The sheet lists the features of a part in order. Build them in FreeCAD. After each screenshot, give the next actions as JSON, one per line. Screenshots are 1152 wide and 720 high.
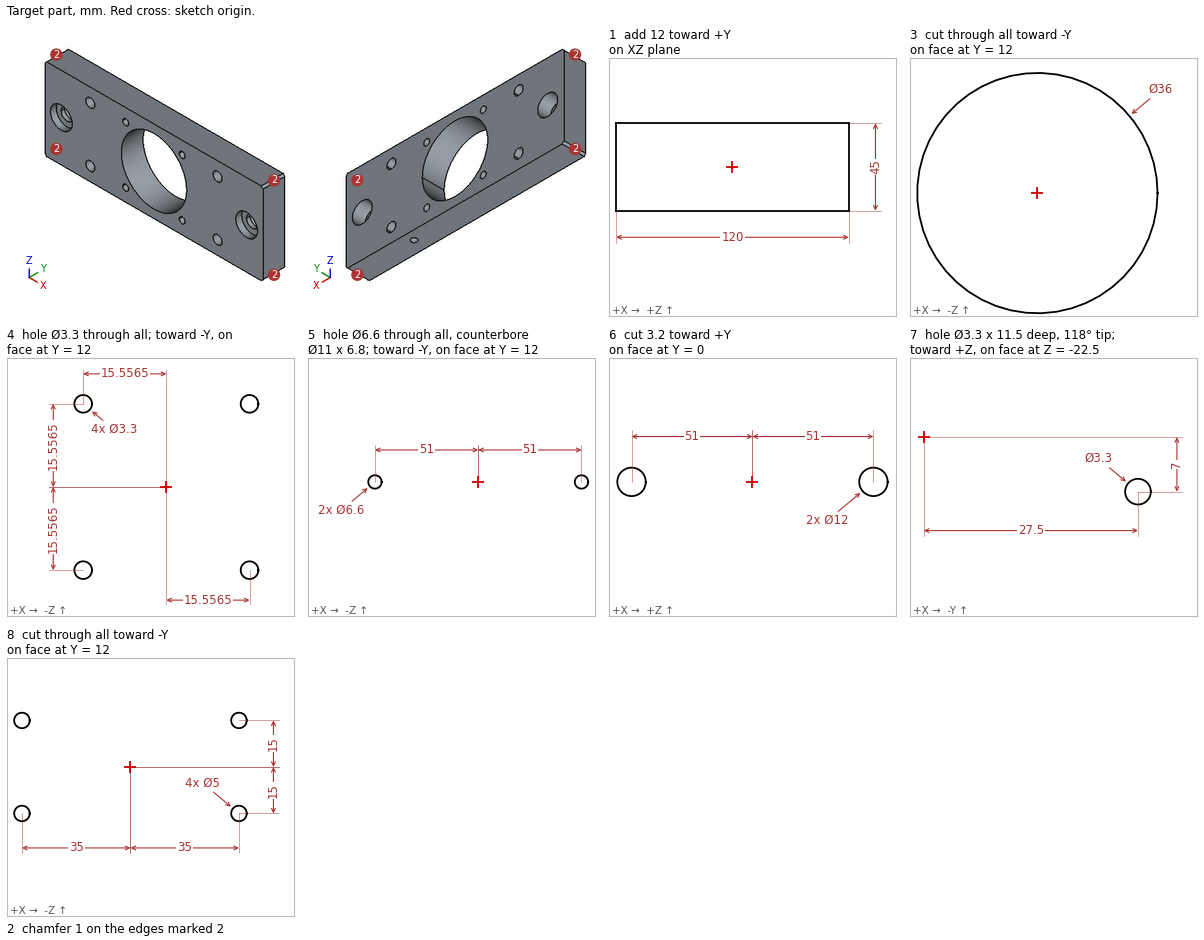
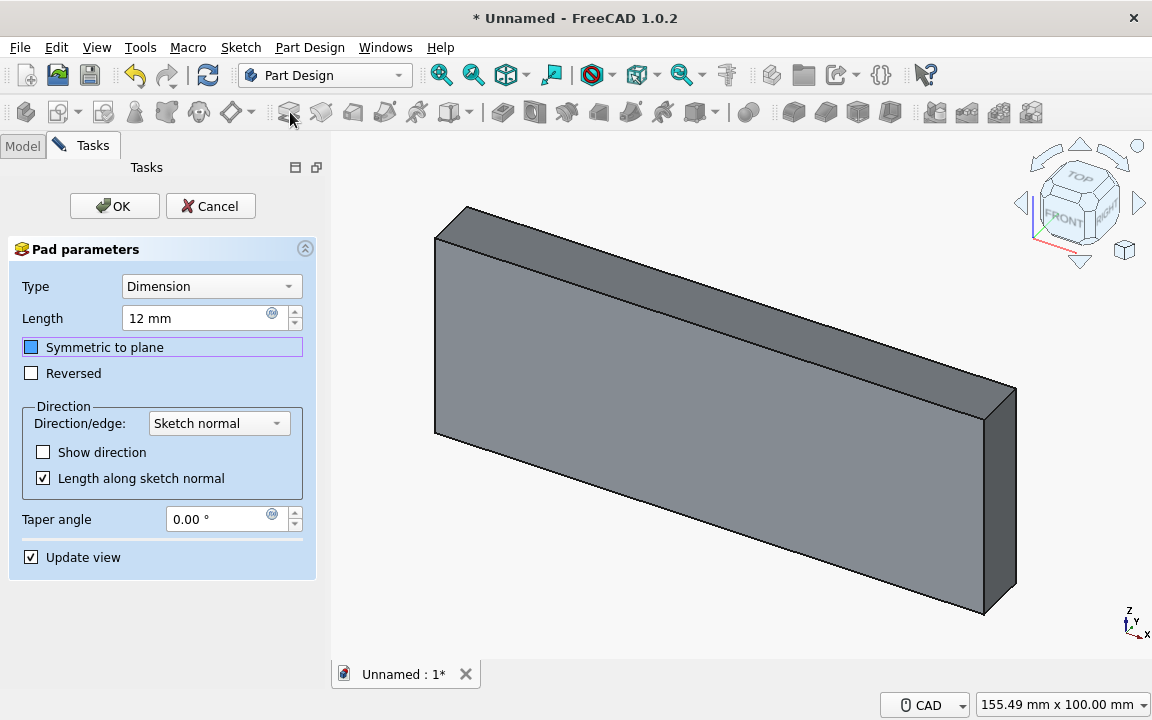
{"action": "left_click", "coordinate": [30, 373]}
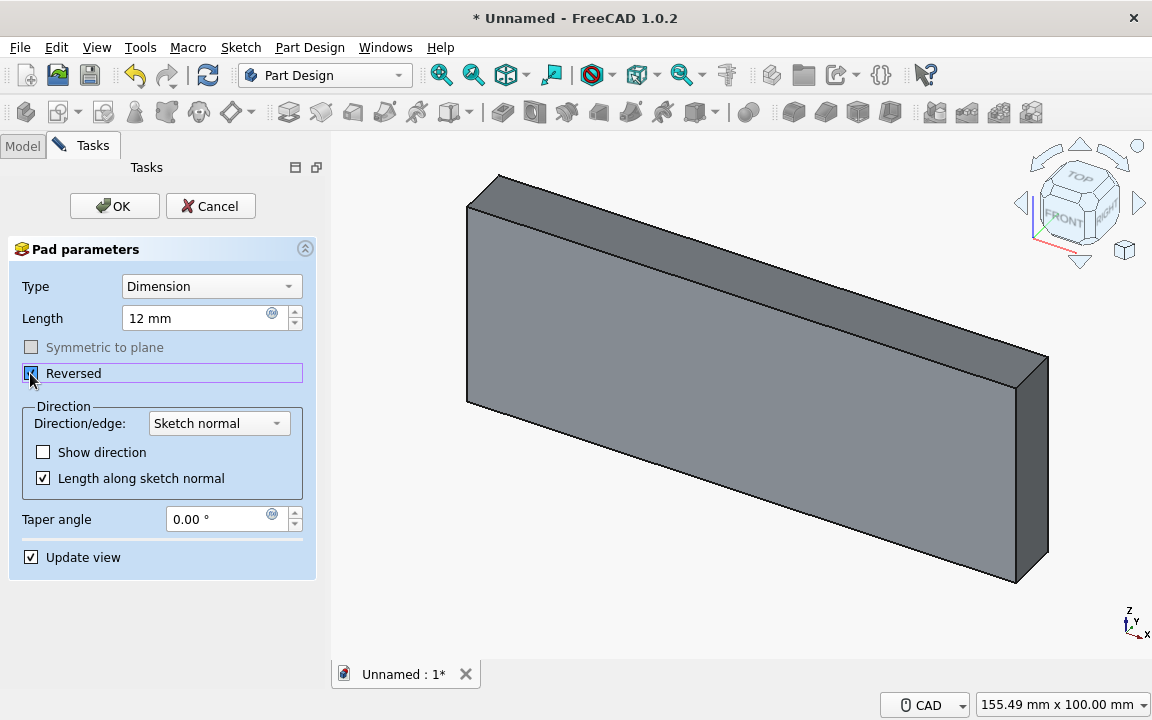
{"action": "left_click", "coordinate": [115, 206]}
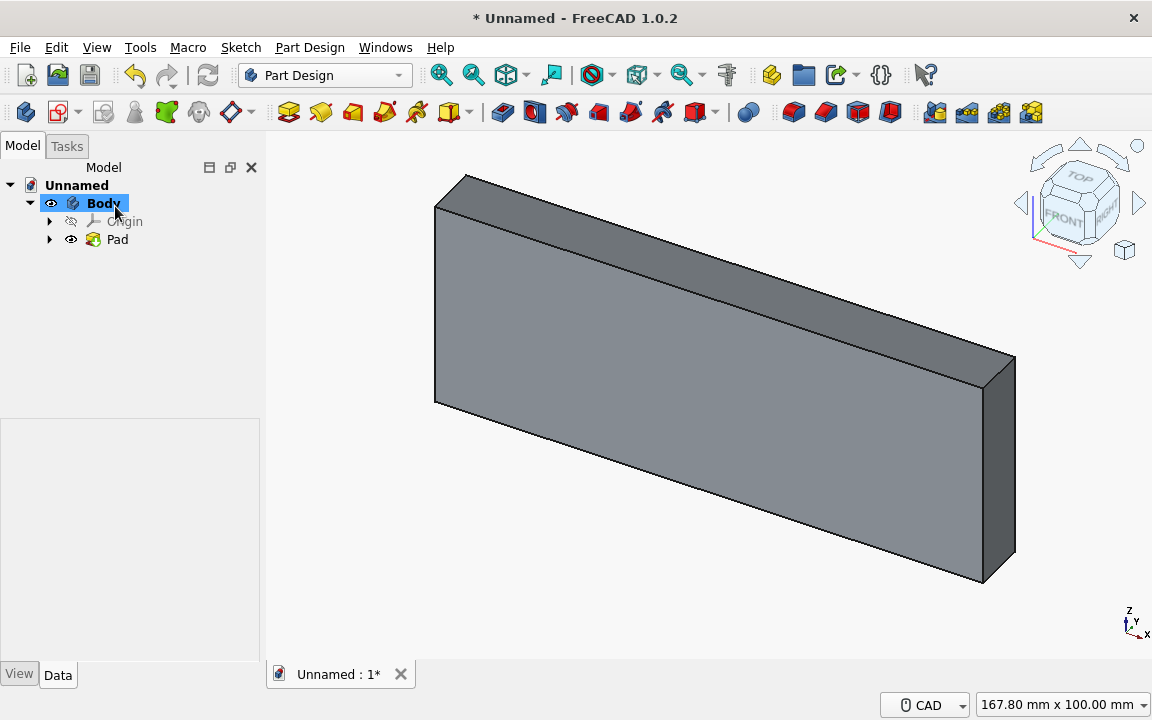
{"action": "left_click", "coordinate": [999, 372]}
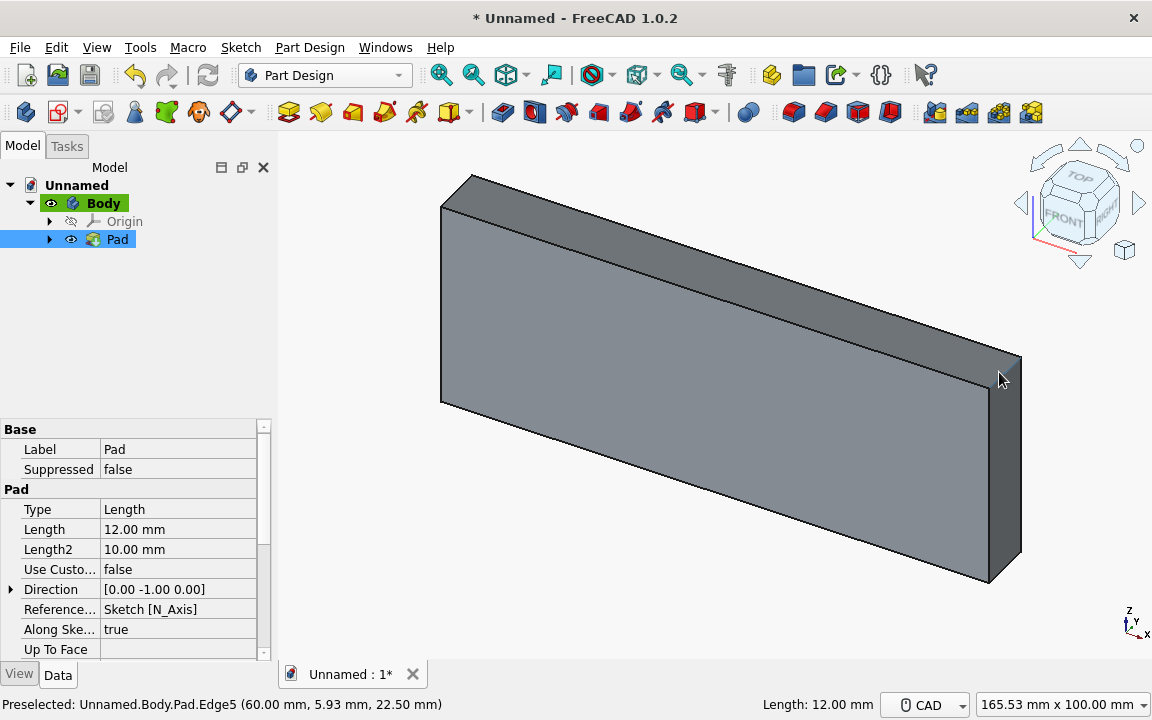
{"action": "key", "text": "0"}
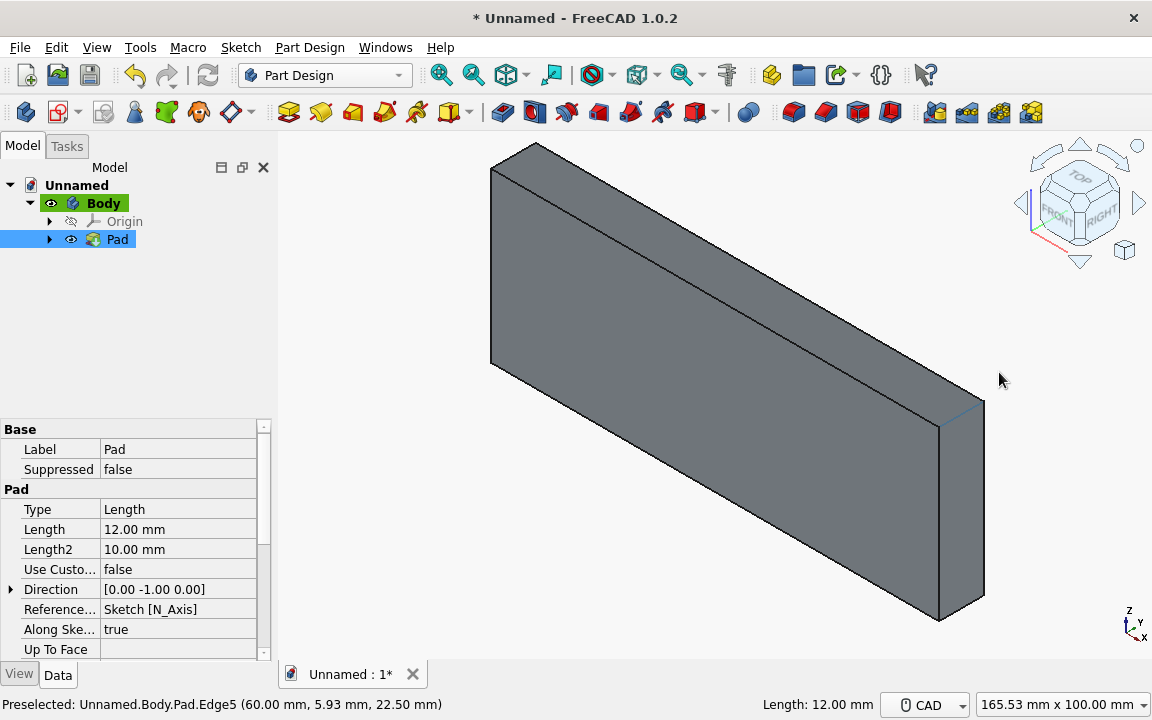
{"action": "key", "text": "2"}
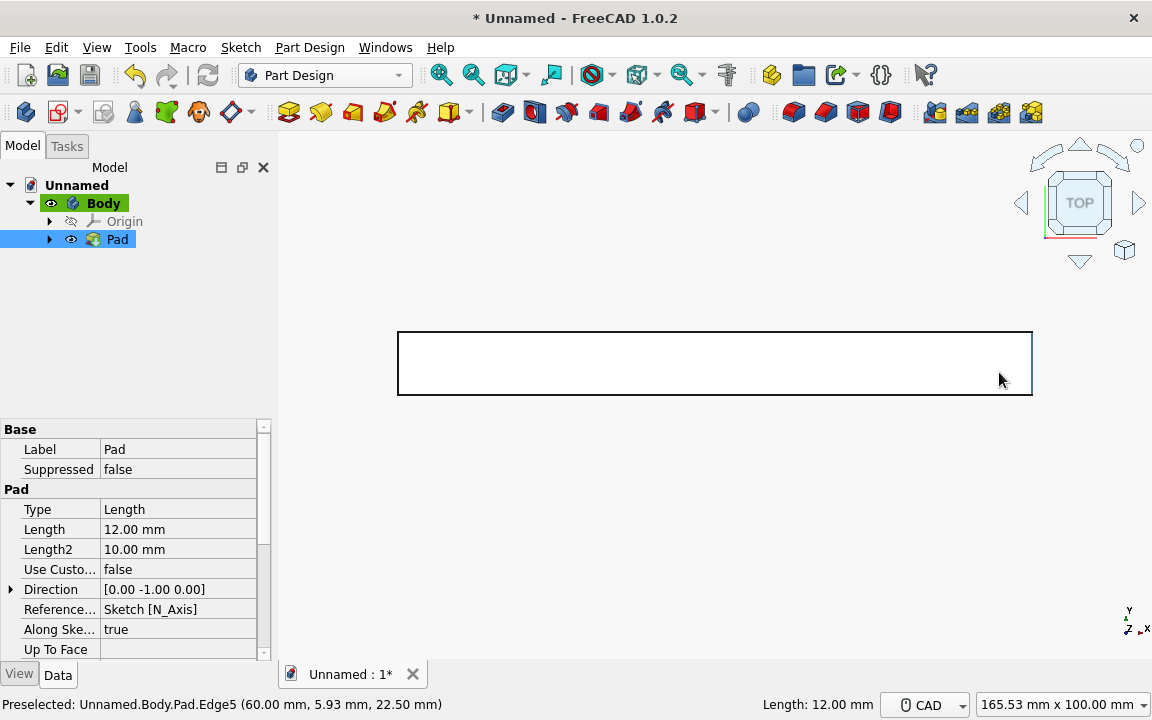
{"action": "left_click", "coordinate": [398, 362], "text": "ctrl"}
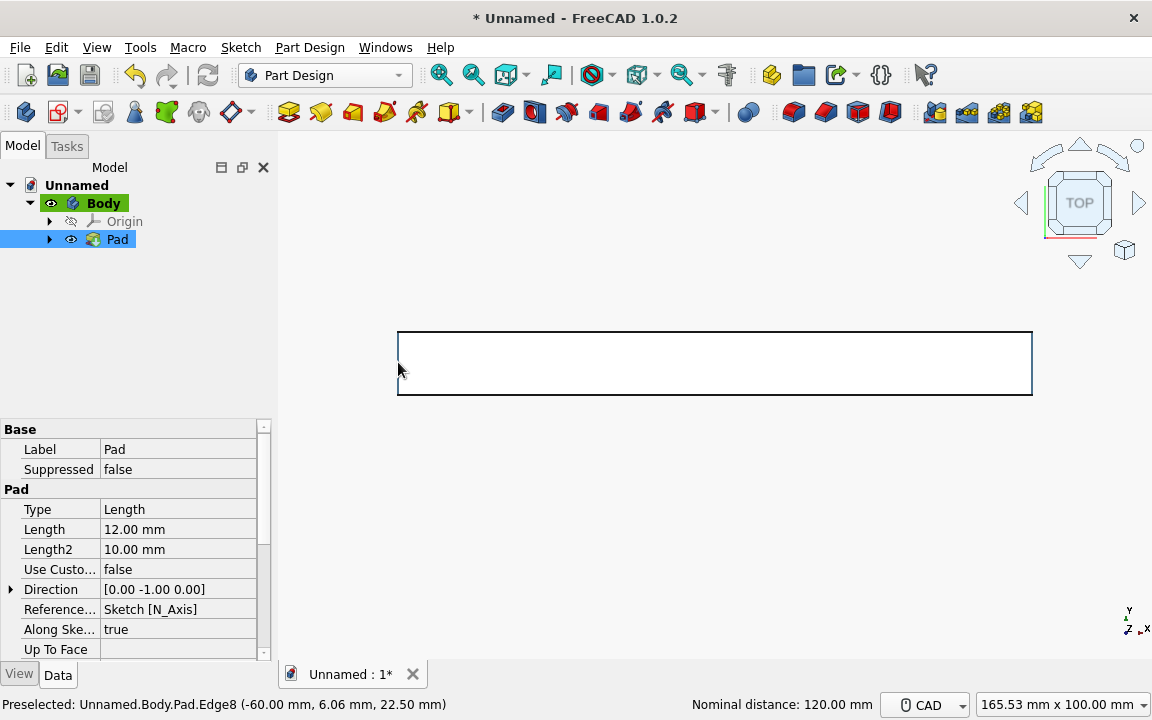
{"action": "key", "text": "1"}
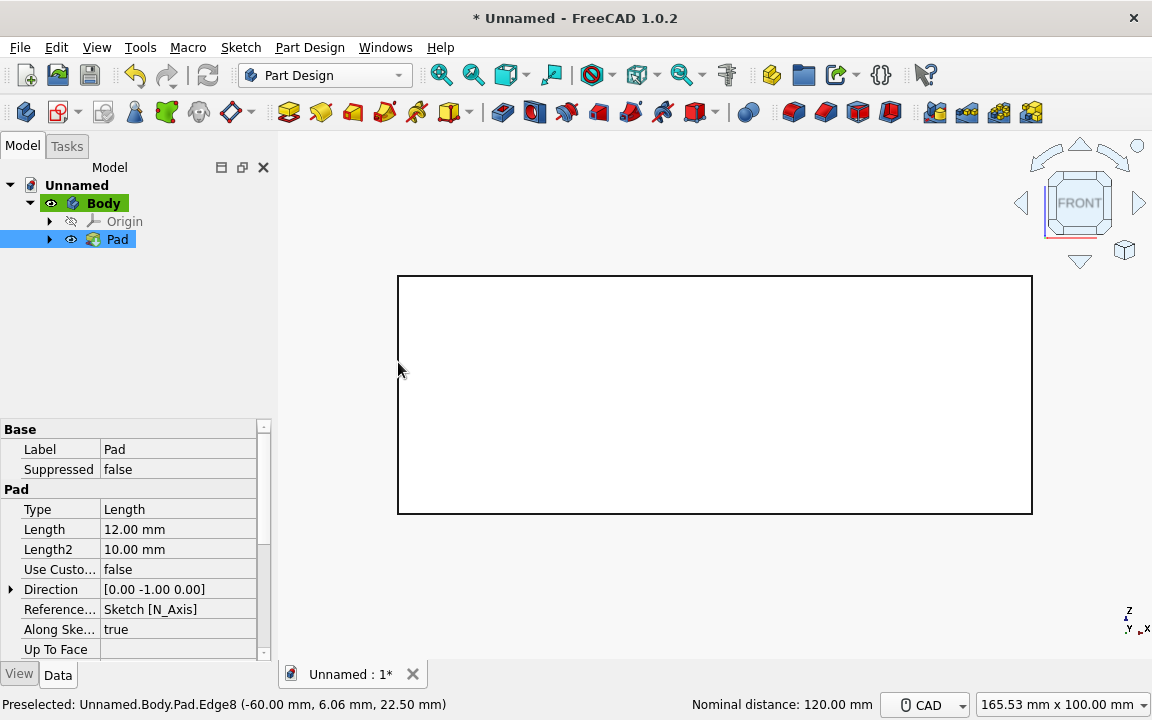
{"action": "key", "text": "3"}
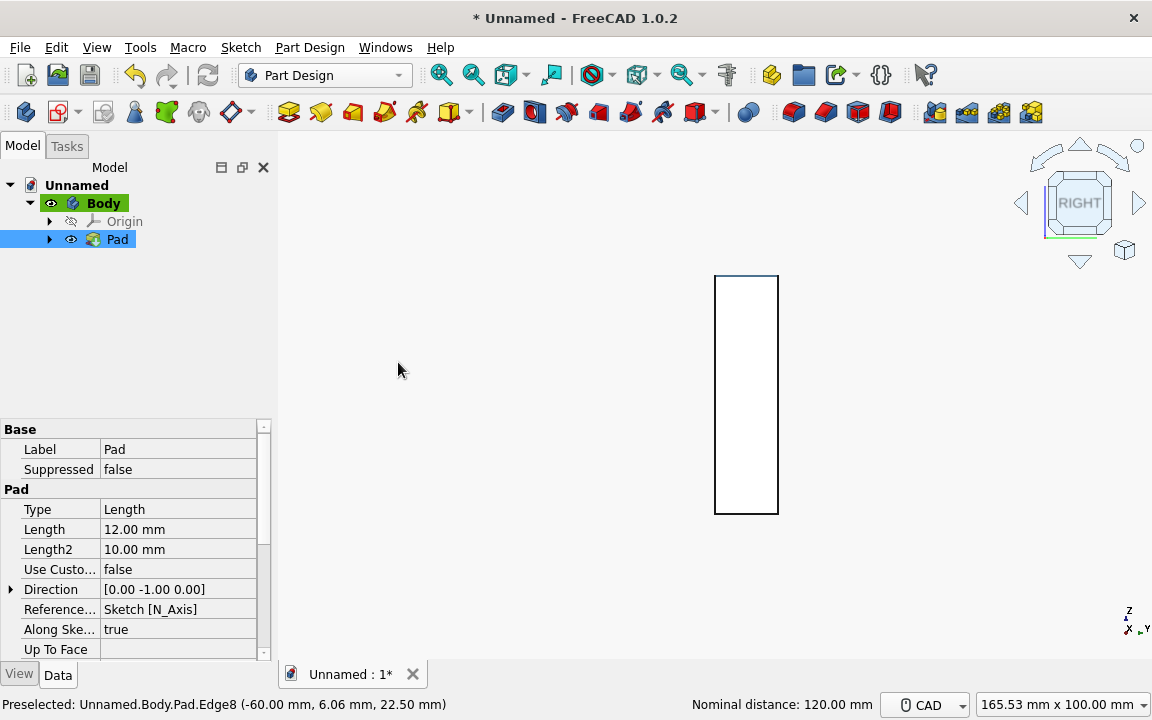
{"action": "left_click", "coordinate": [747, 513], "text": "ctrl"}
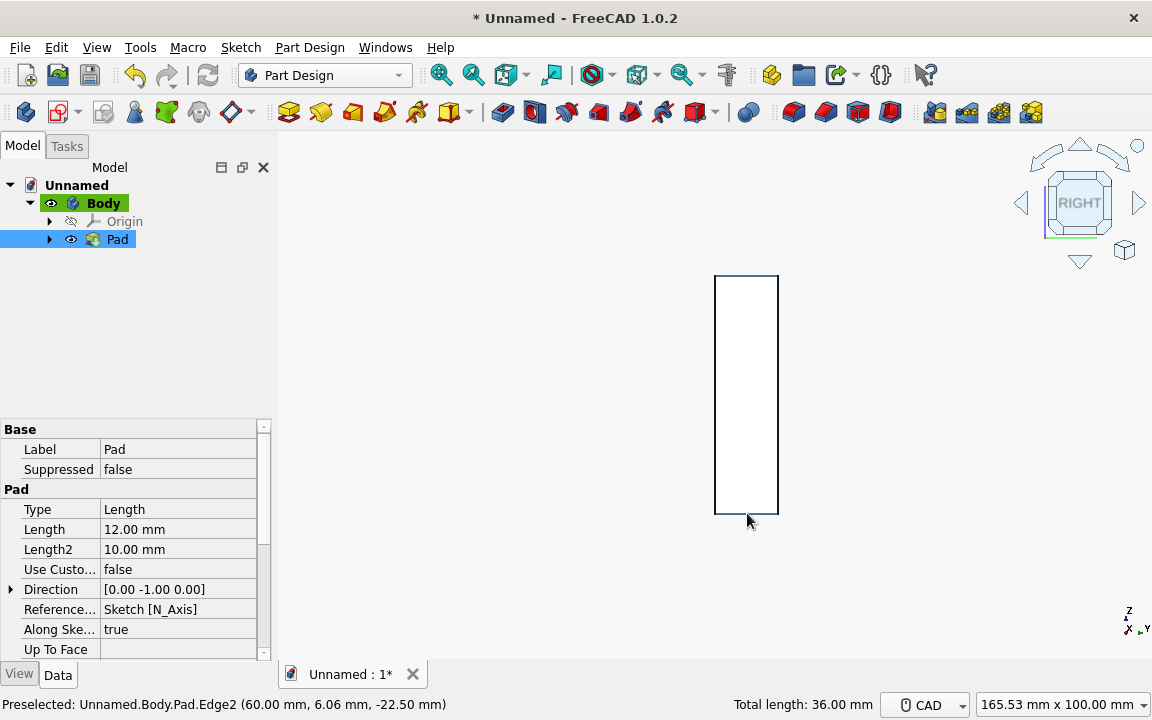
{"action": "key", "text": "5"}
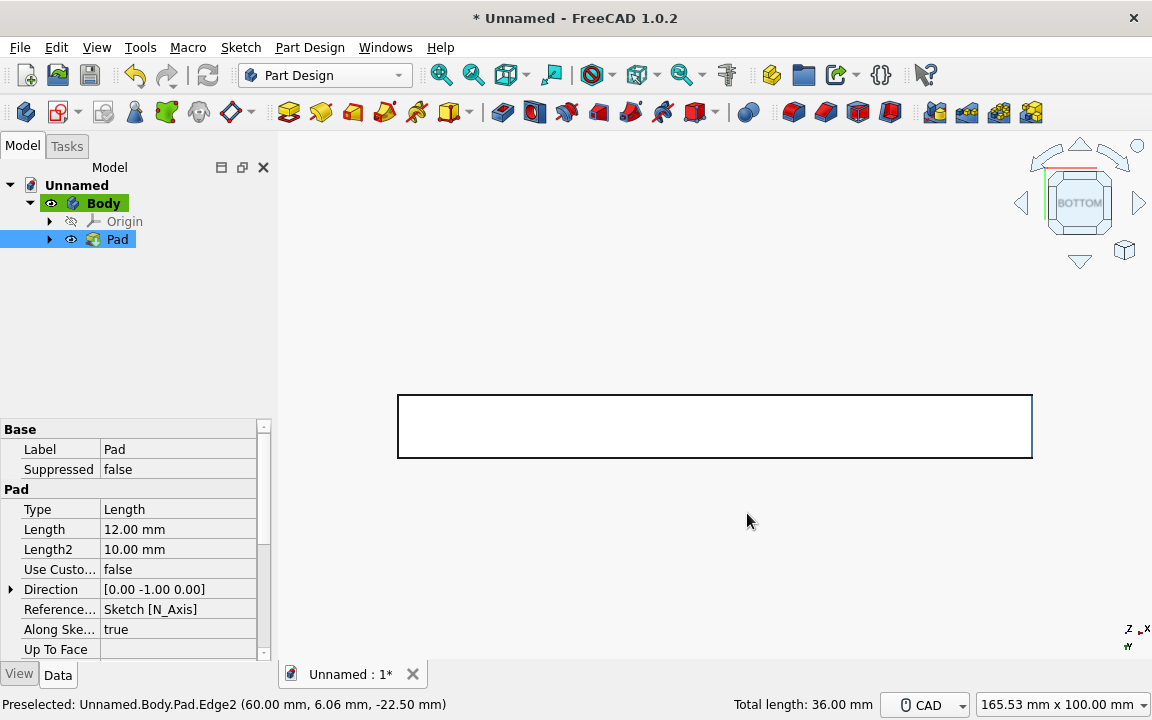
{"action": "left_click", "coordinate": [398, 426], "text": "ctrl"}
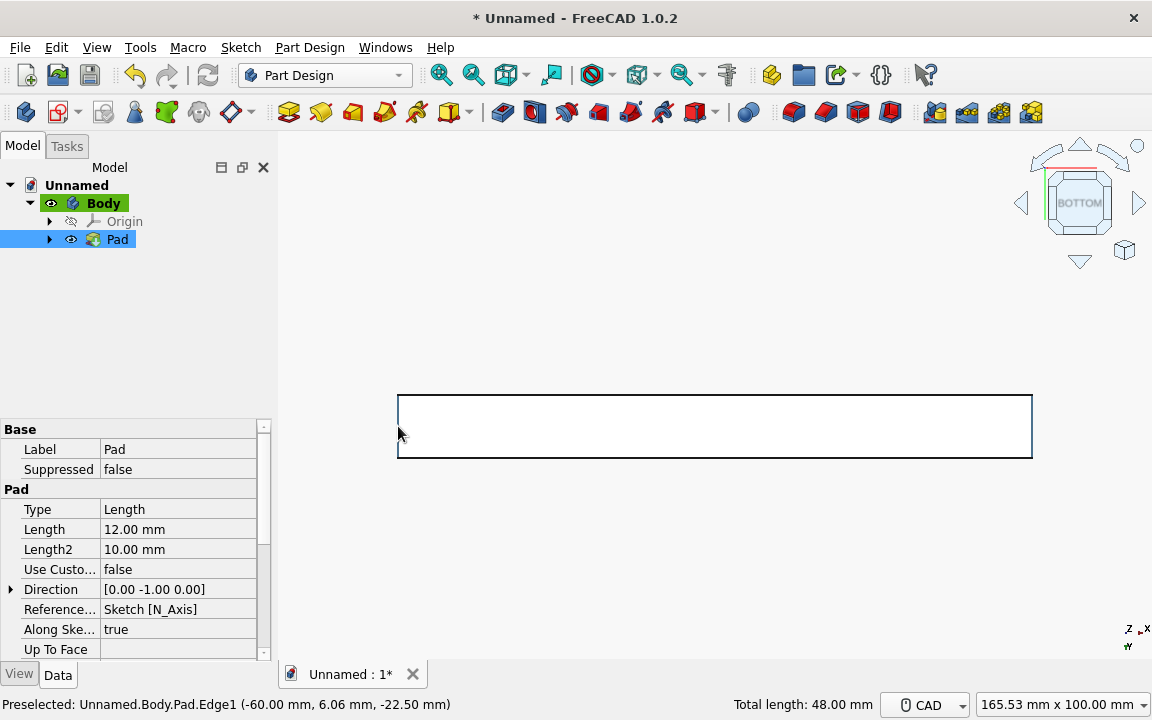
{"action": "left_click", "coordinate": [826, 112]}